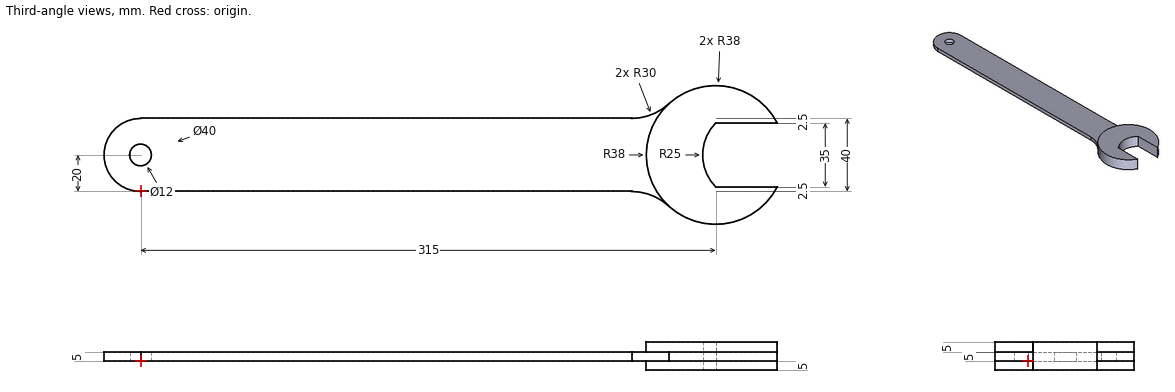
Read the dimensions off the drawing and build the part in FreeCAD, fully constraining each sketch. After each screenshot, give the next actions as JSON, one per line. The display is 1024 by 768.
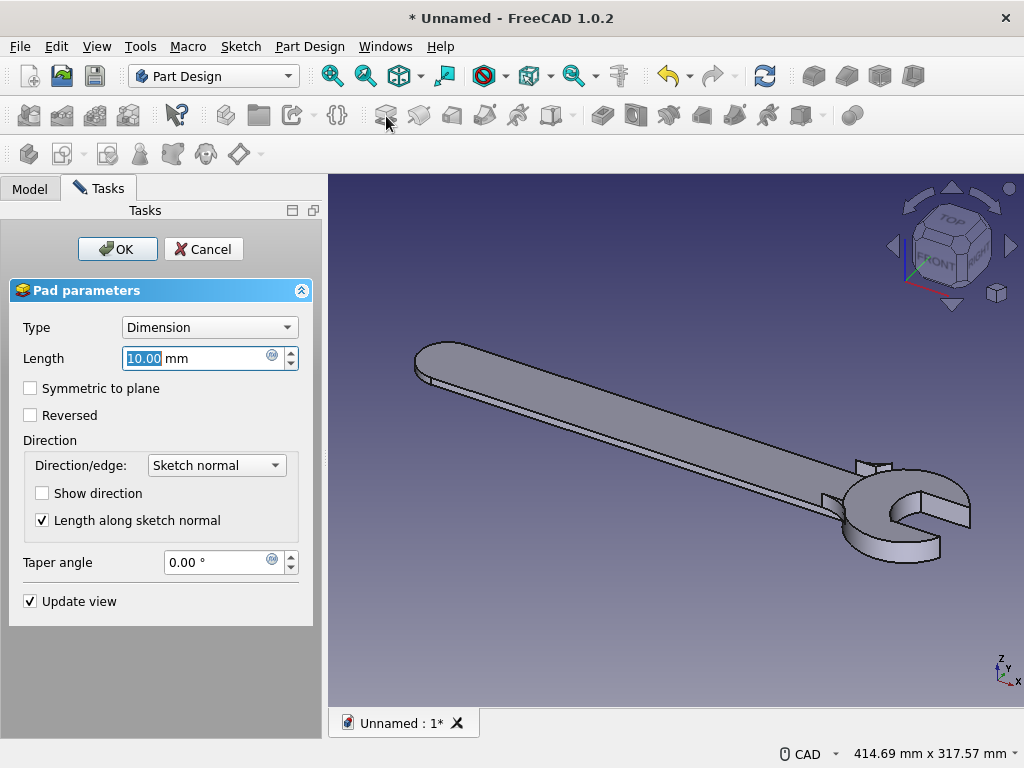
{"action": "type", "text": "5"}
{"action": "key", "text": "Tab"}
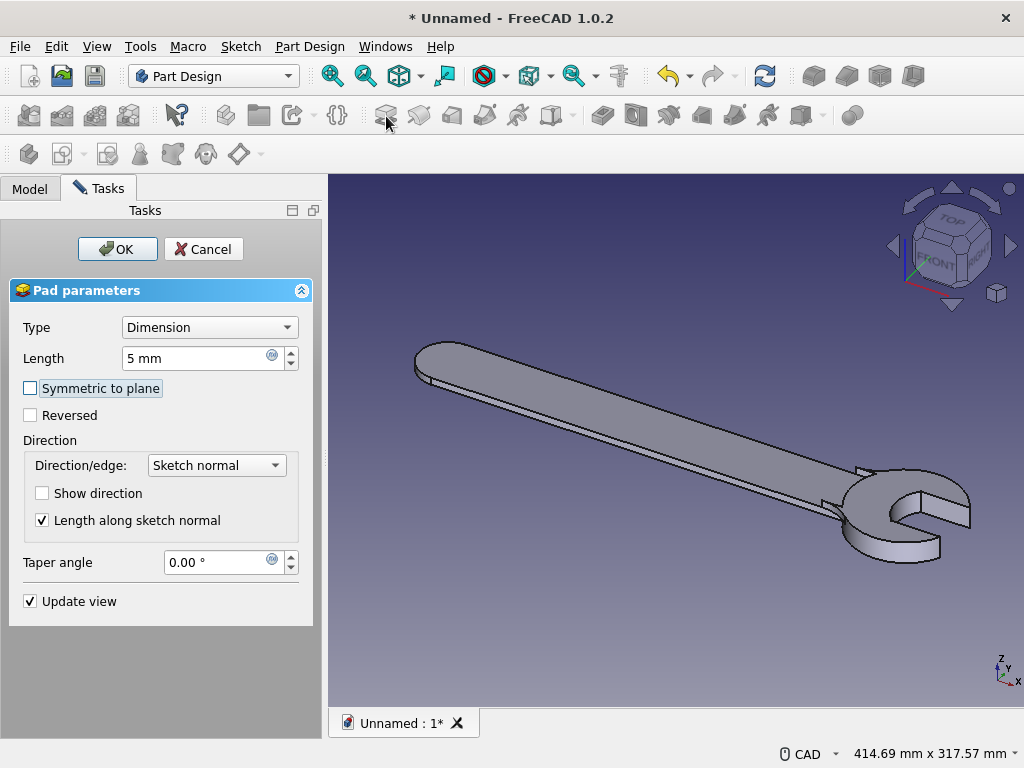
{"action": "left_click", "coordinate": [31, 415]}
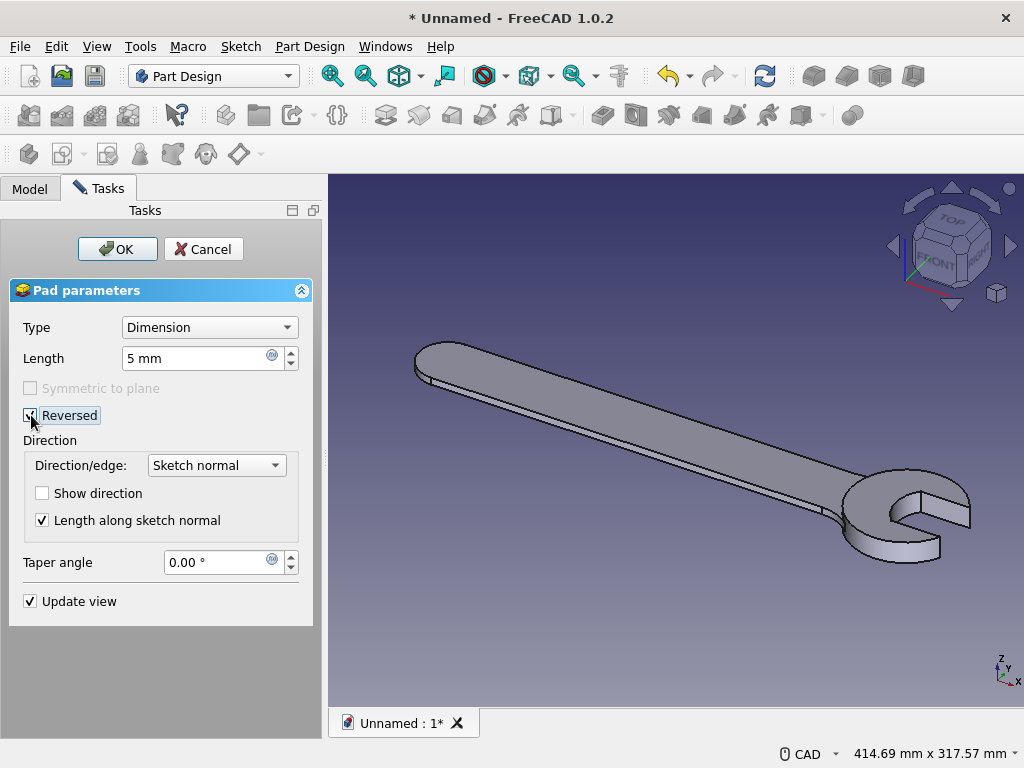
{"action": "left_click", "coordinate": [118, 249]}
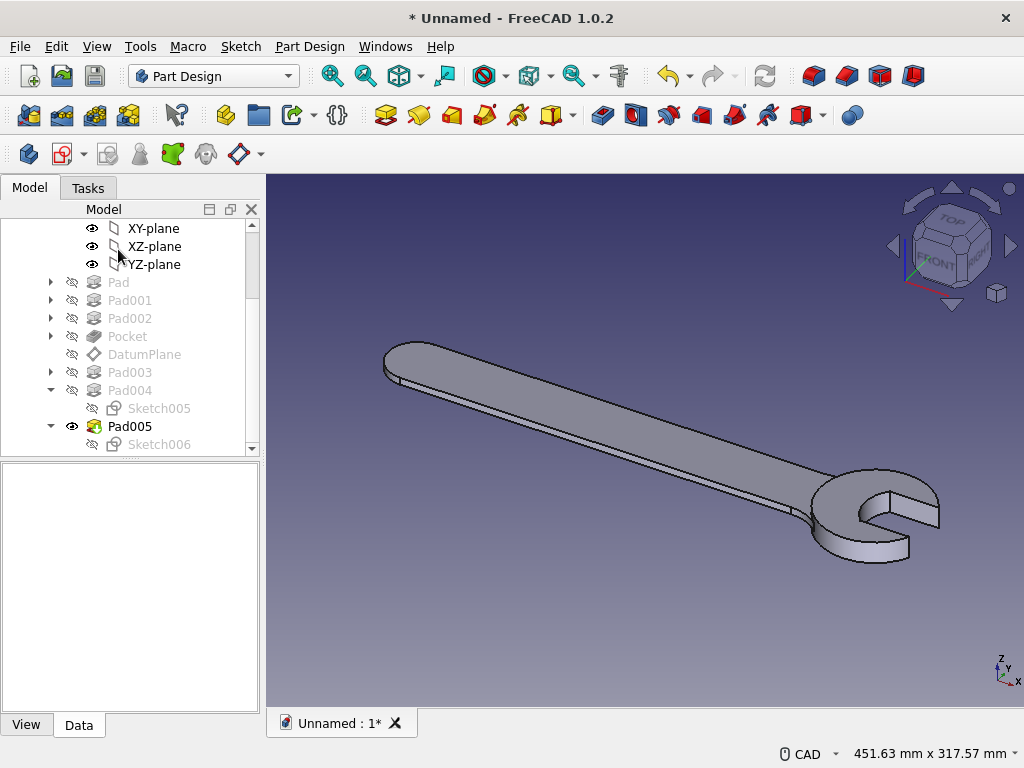
{"action": "left_click", "coordinate": [62, 154]}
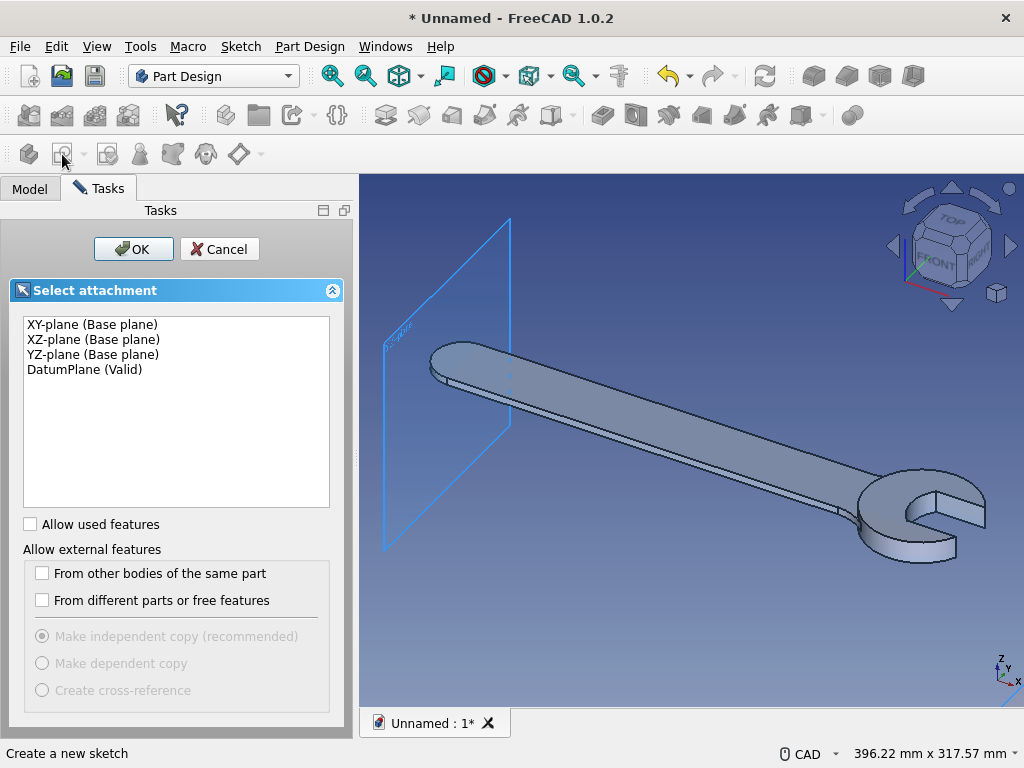
{"action": "left_click", "coordinate": [84, 324]}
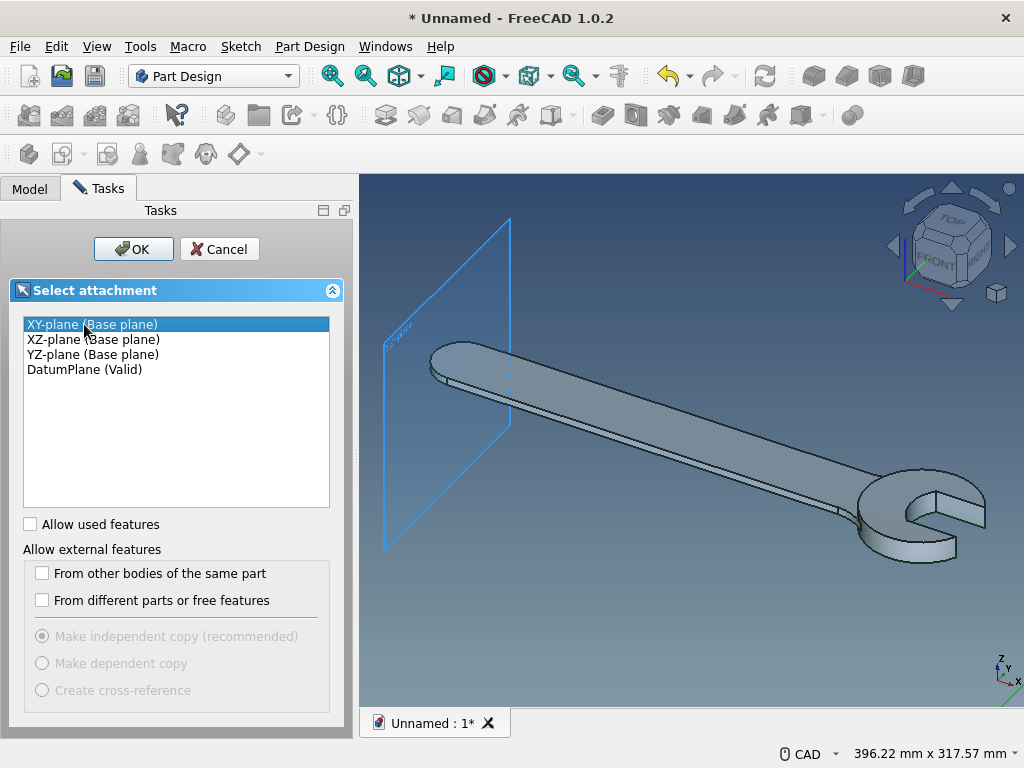
{"action": "left_click", "coordinate": [134, 249]}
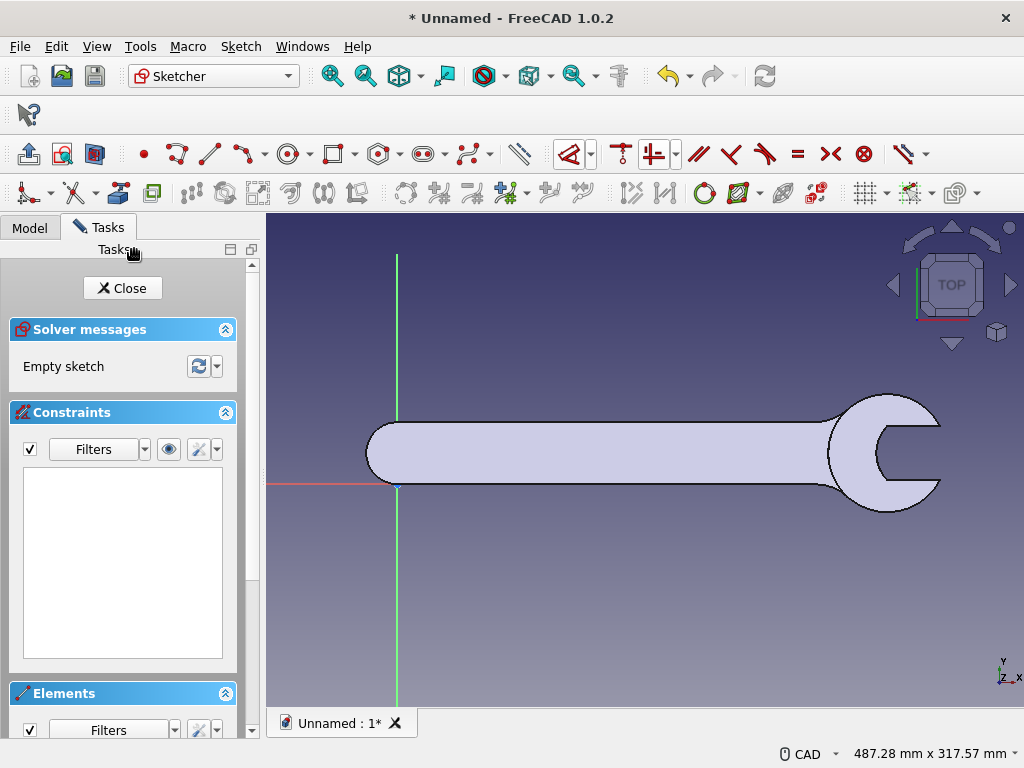
{"action": "left_click", "coordinate": [95, 154]}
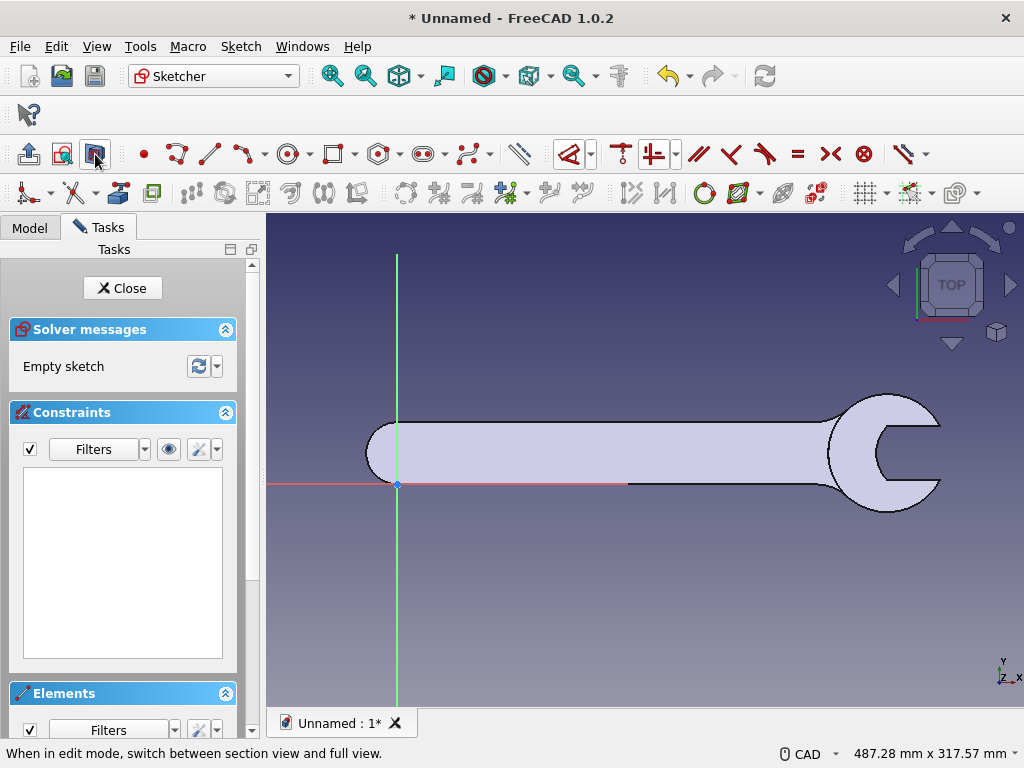
{"action": "scroll", "coordinate": [369, 465], "scroll_direction": "up", "scroll_amount": 10}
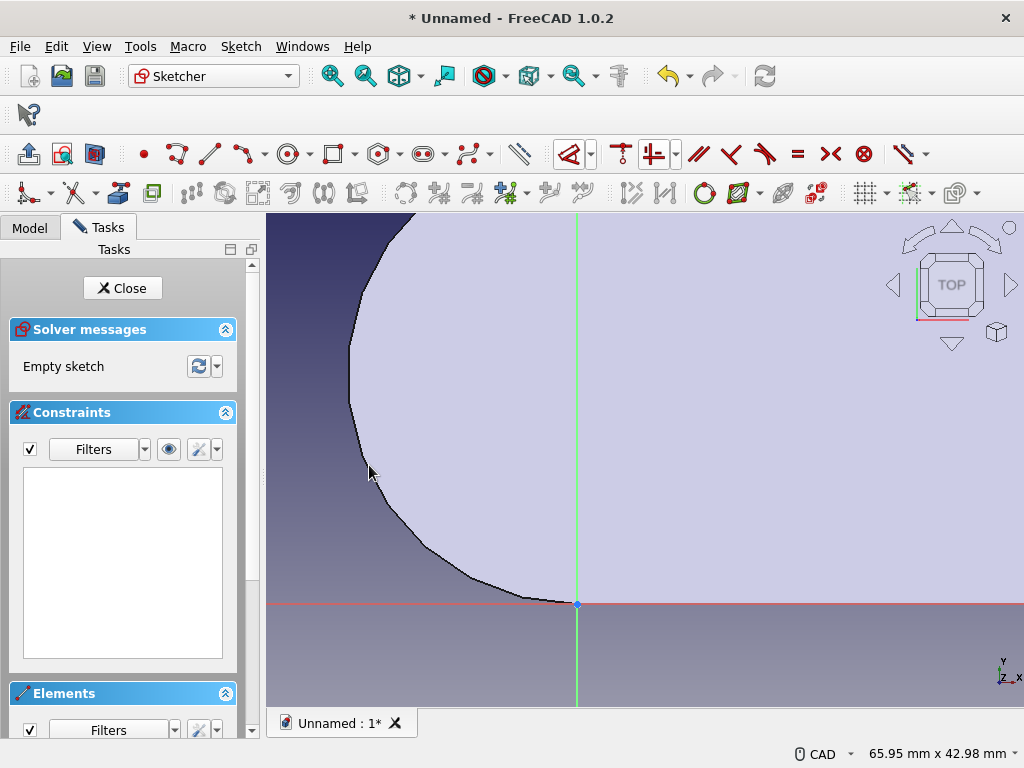
{"action": "left_click", "coordinate": [288, 154]}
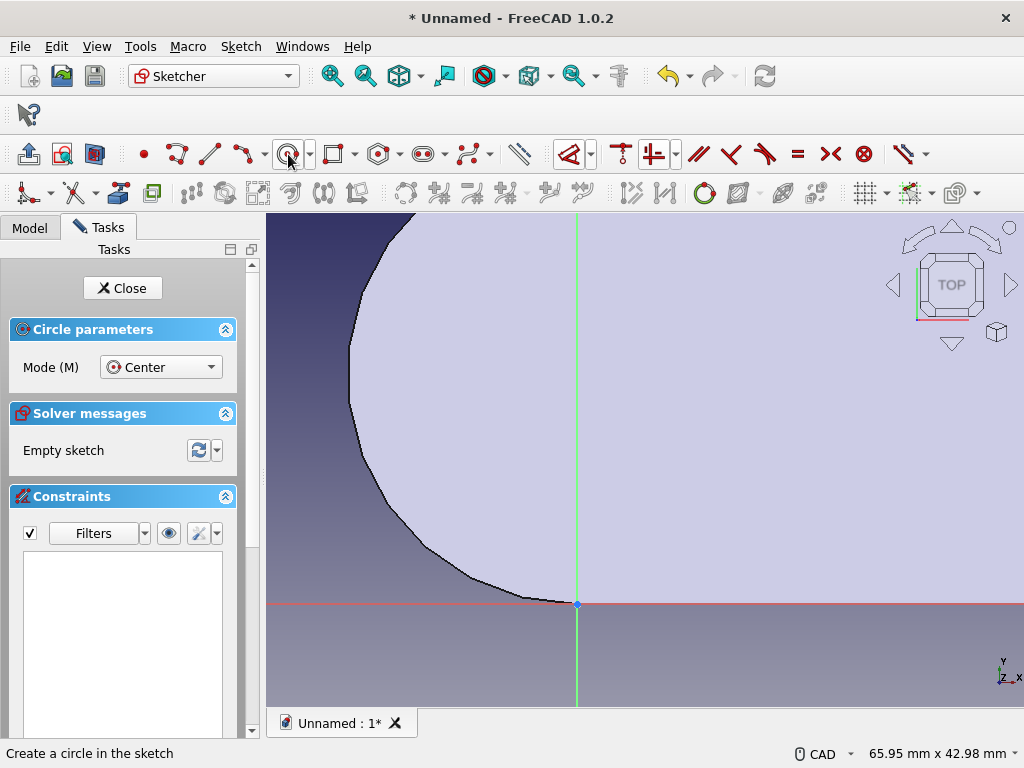
{"action": "left_click", "coordinate": [577, 374]}
{"action": "mouse_move", "coordinate": [626, 326]}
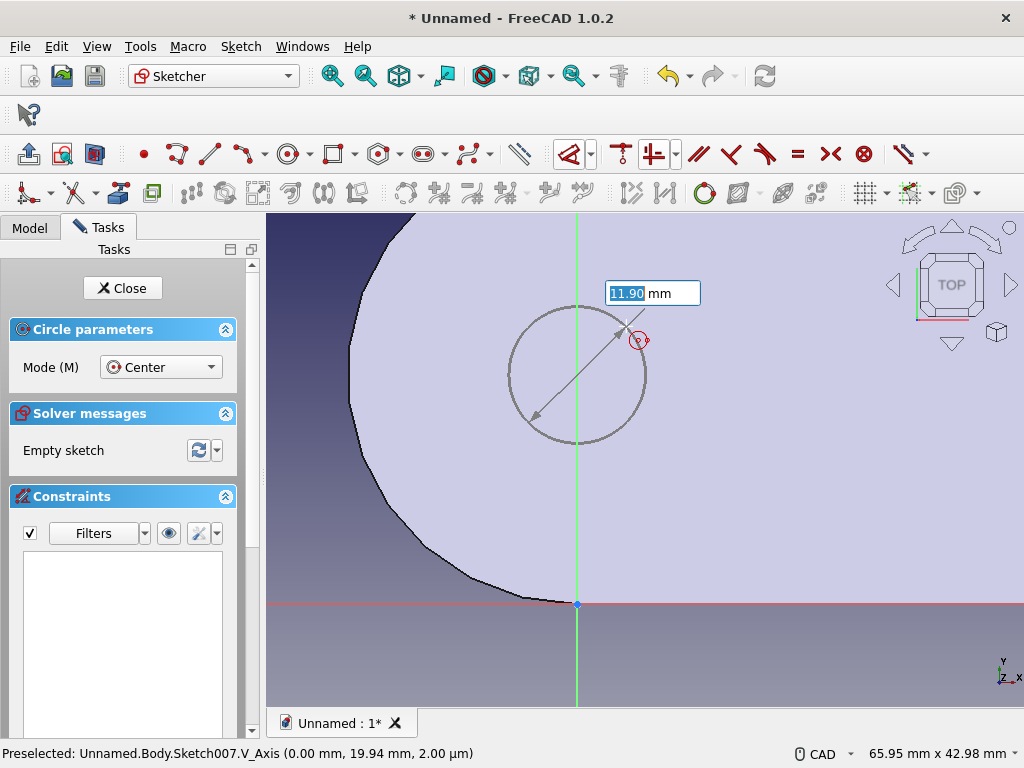
{"action": "type", "text": "12"}
{"action": "key", "text": "Return"}
{"action": "key", "text": "Escape"}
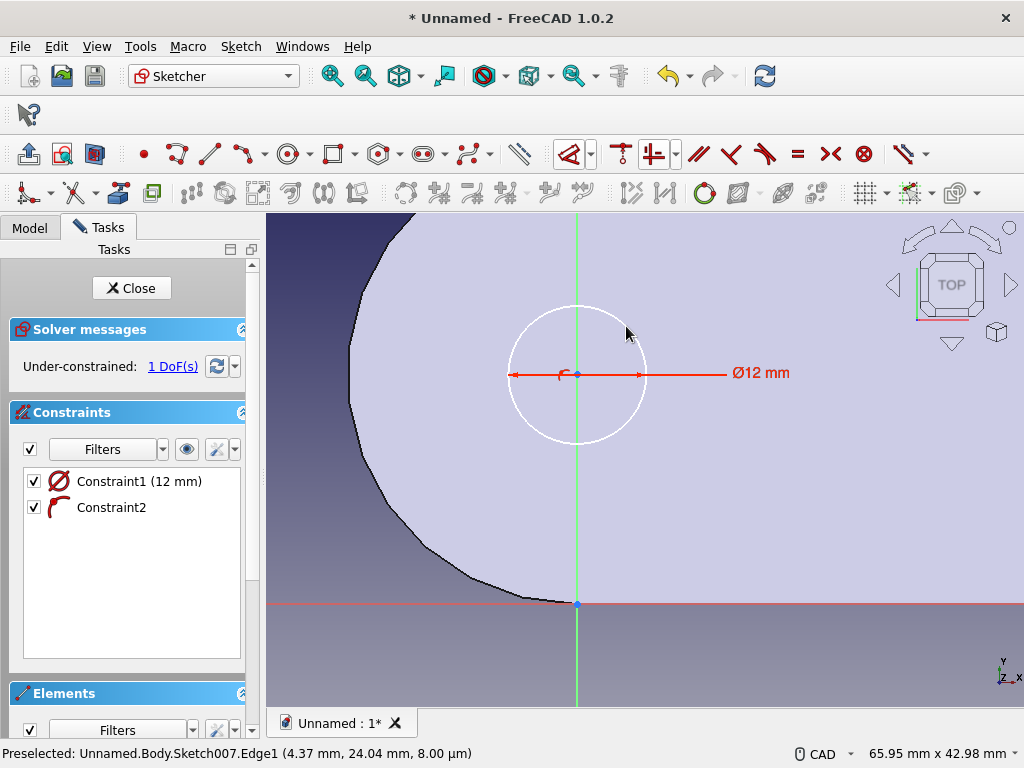
{"action": "left_click", "coordinate": [577, 375]}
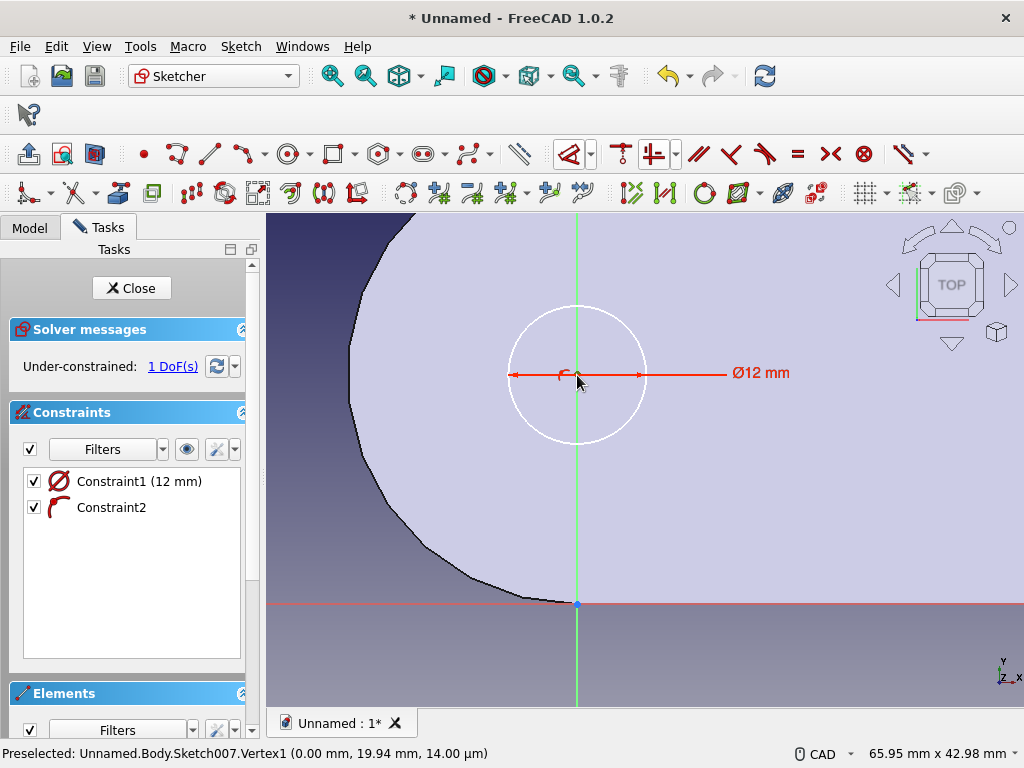
{"action": "key", "text": "i"}